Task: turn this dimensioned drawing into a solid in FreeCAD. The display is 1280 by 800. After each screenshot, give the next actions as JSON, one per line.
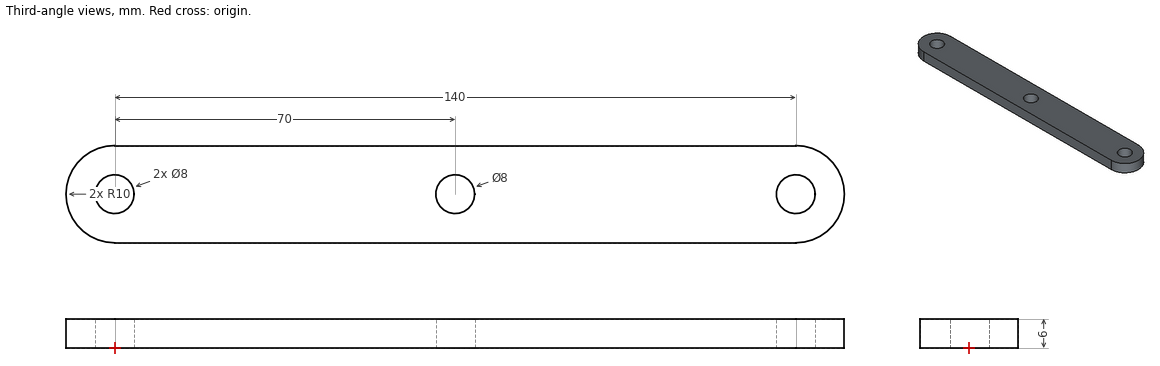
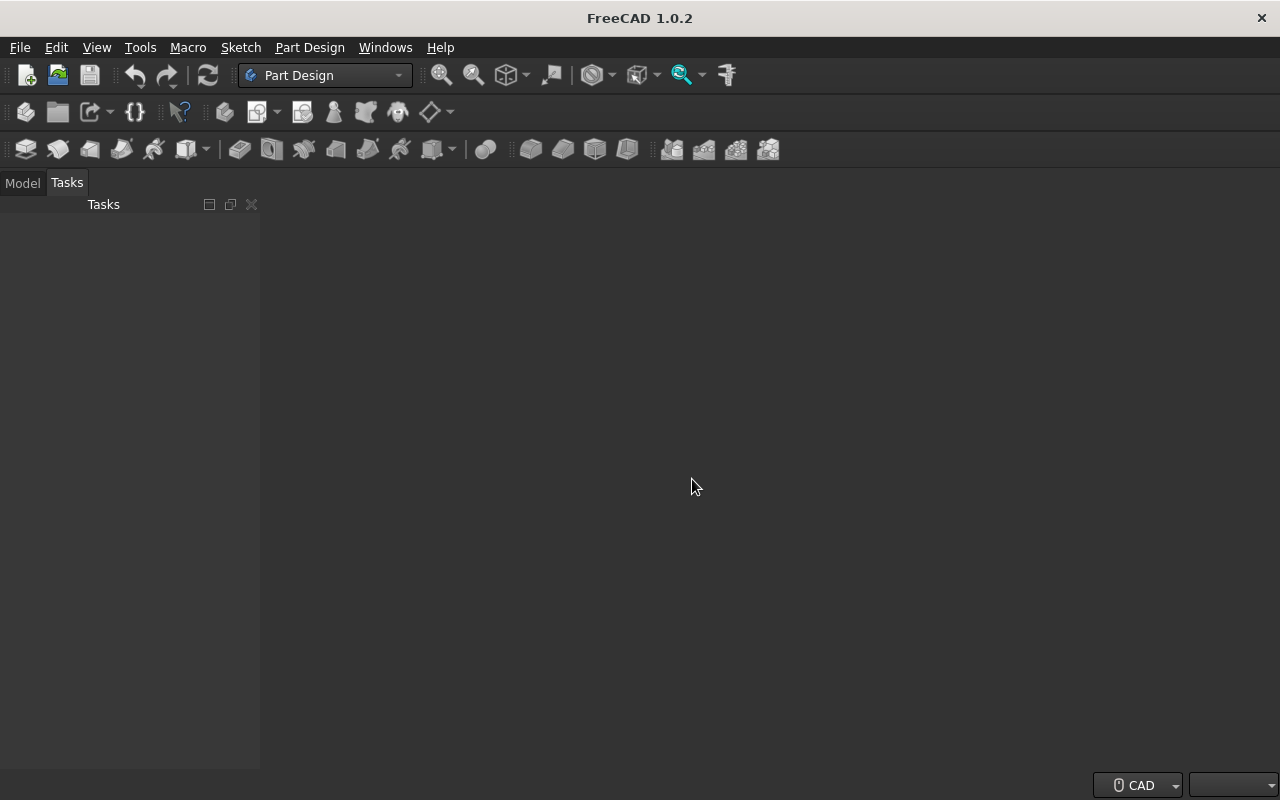
{"action": "left_click", "coordinate": [26, 76]}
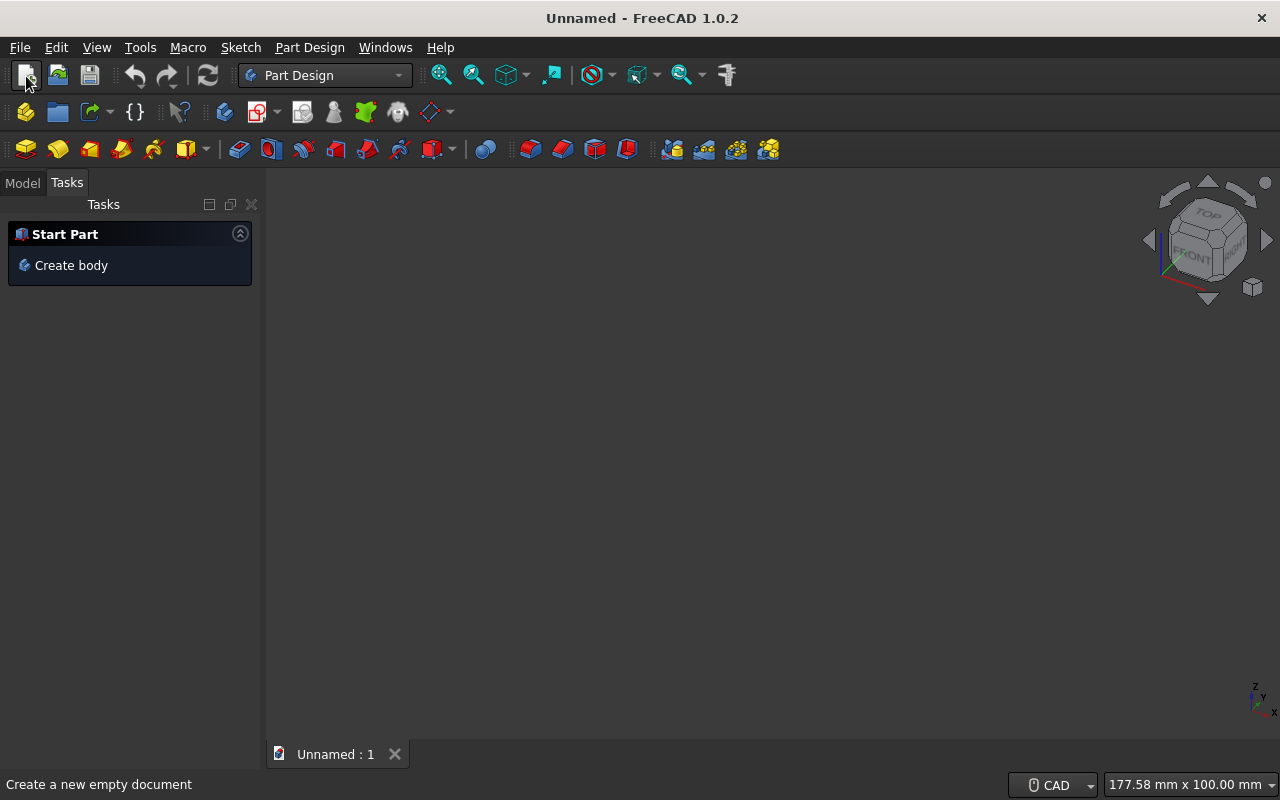
{"action": "left_click", "coordinate": [258, 112]}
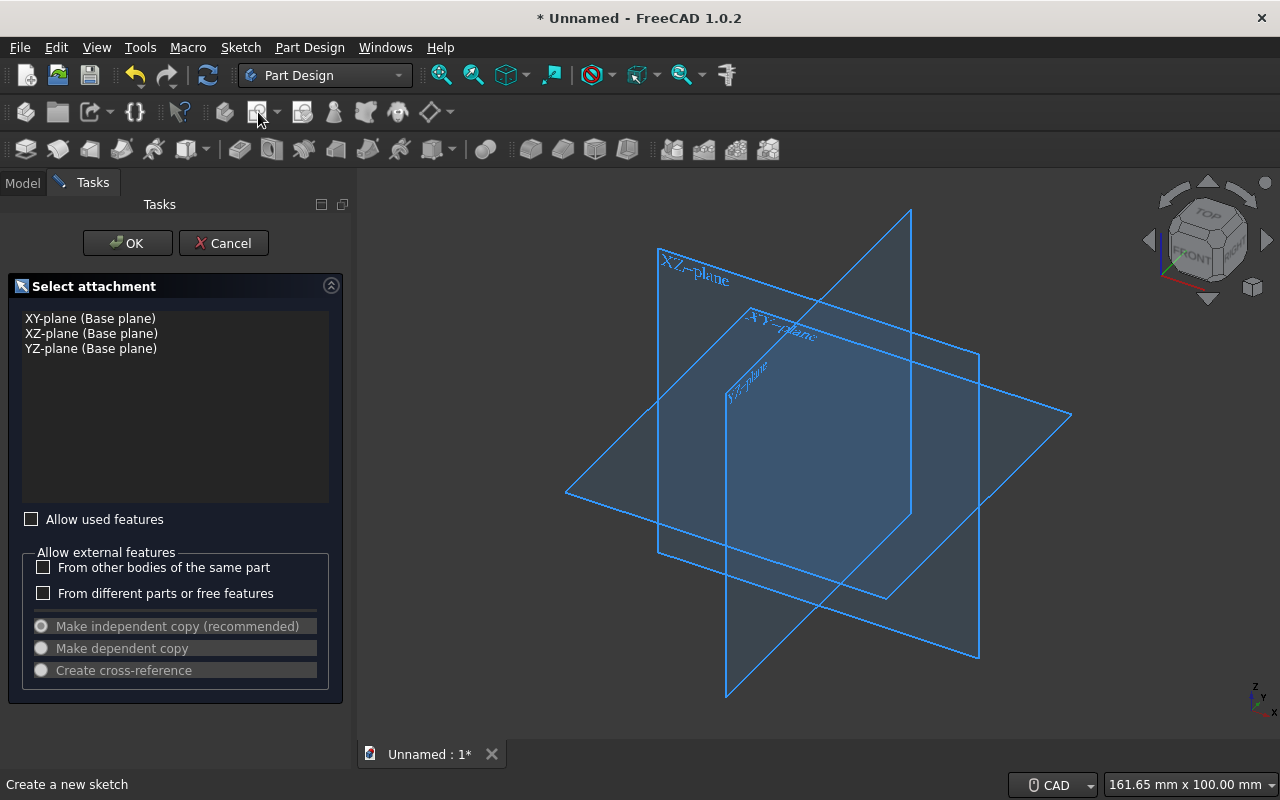
{"action": "left_click", "coordinate": [82, 318]}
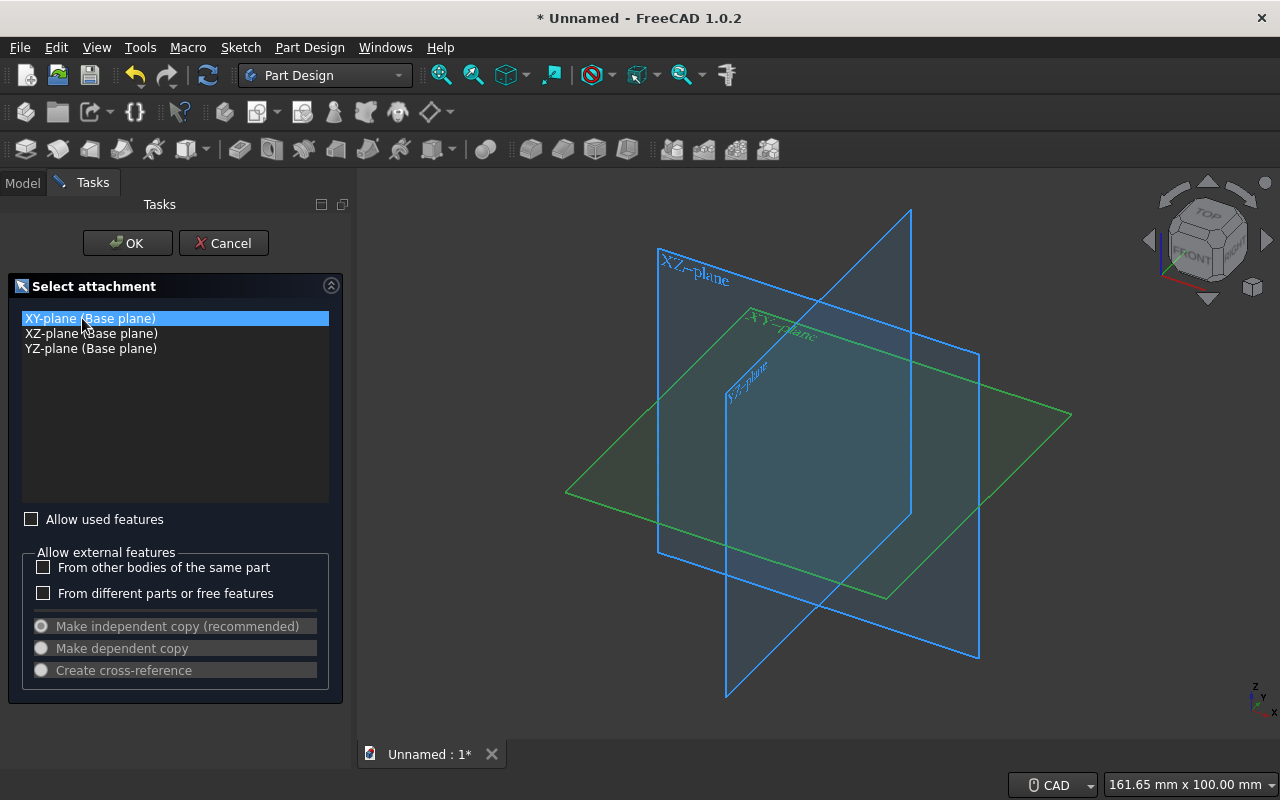
{"action": "left_click", "coordinate": [128, 243]}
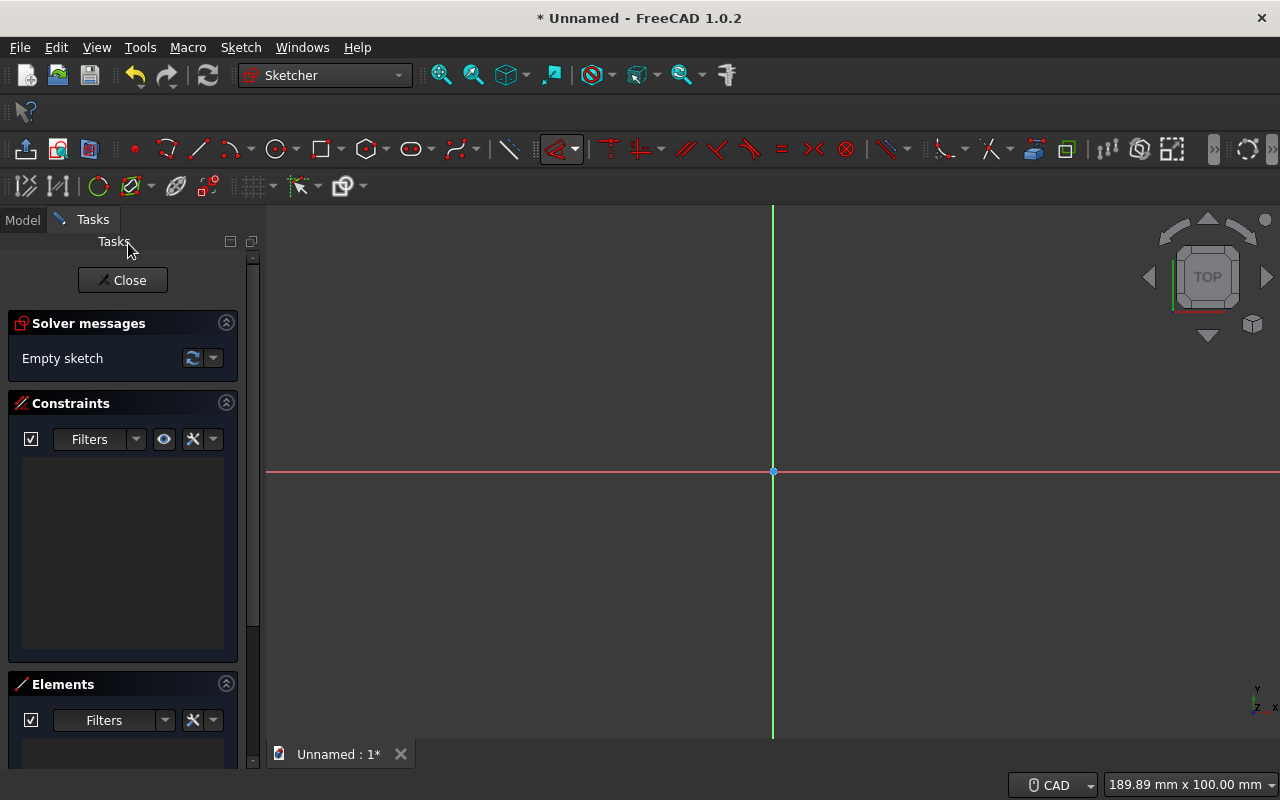
{"action": "scroll", "coordinate": [294, 472], "scroll_direction": "down", "scroll_amount": 3}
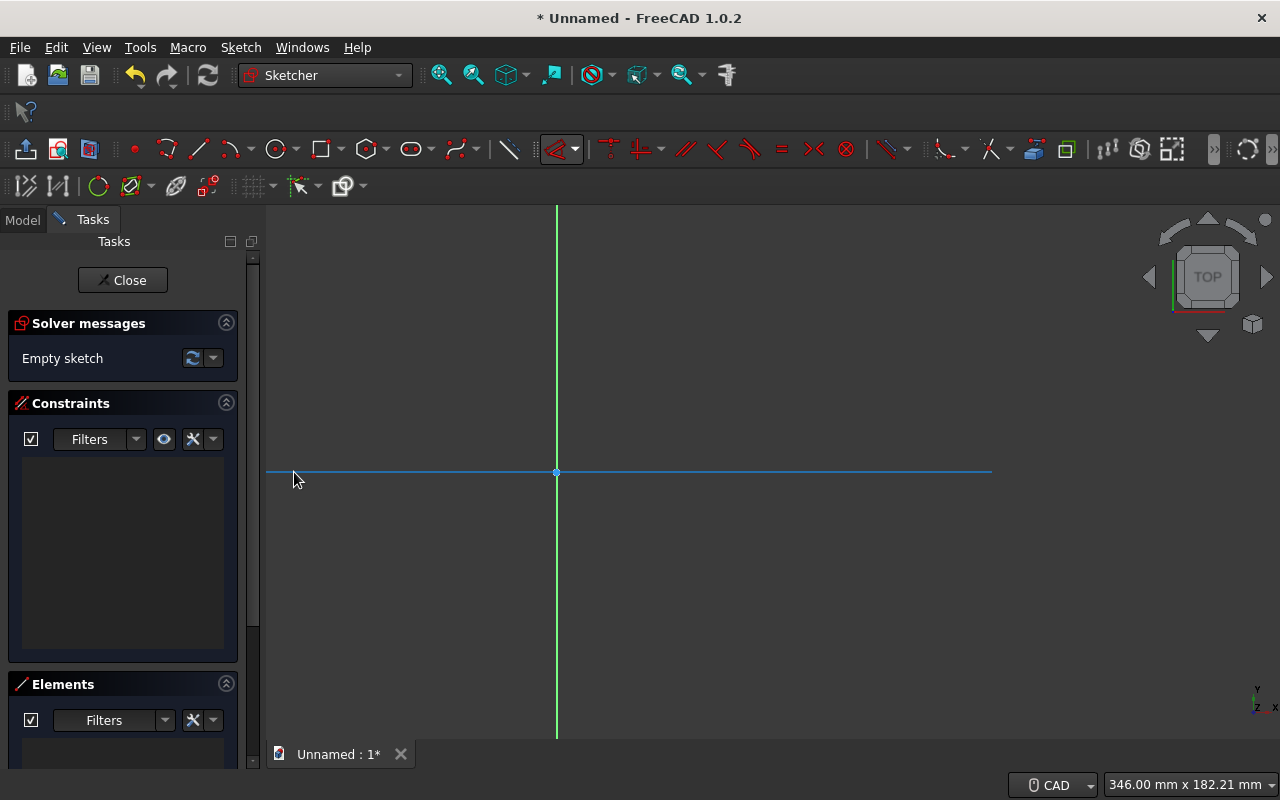
{"action": "key", "text": "g s"}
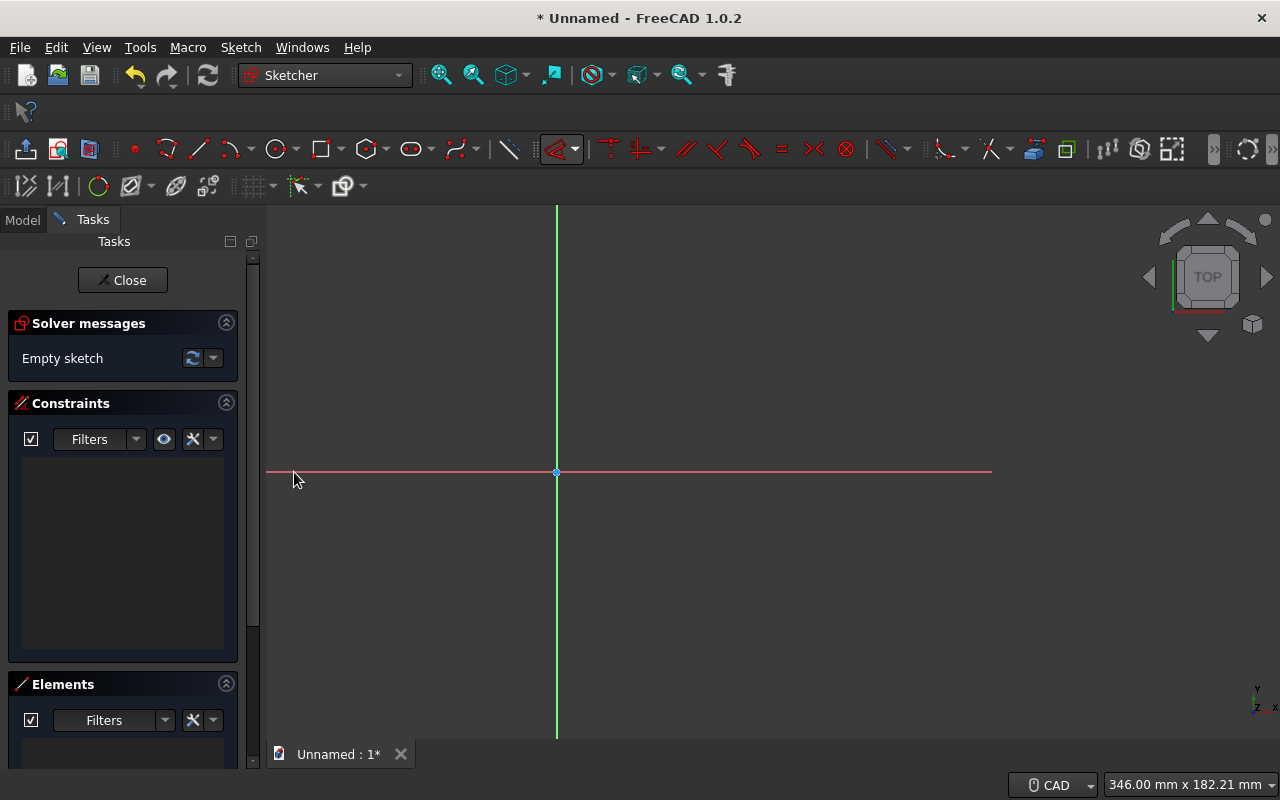
{"action": "left_click", "coordinate": [557, 472]}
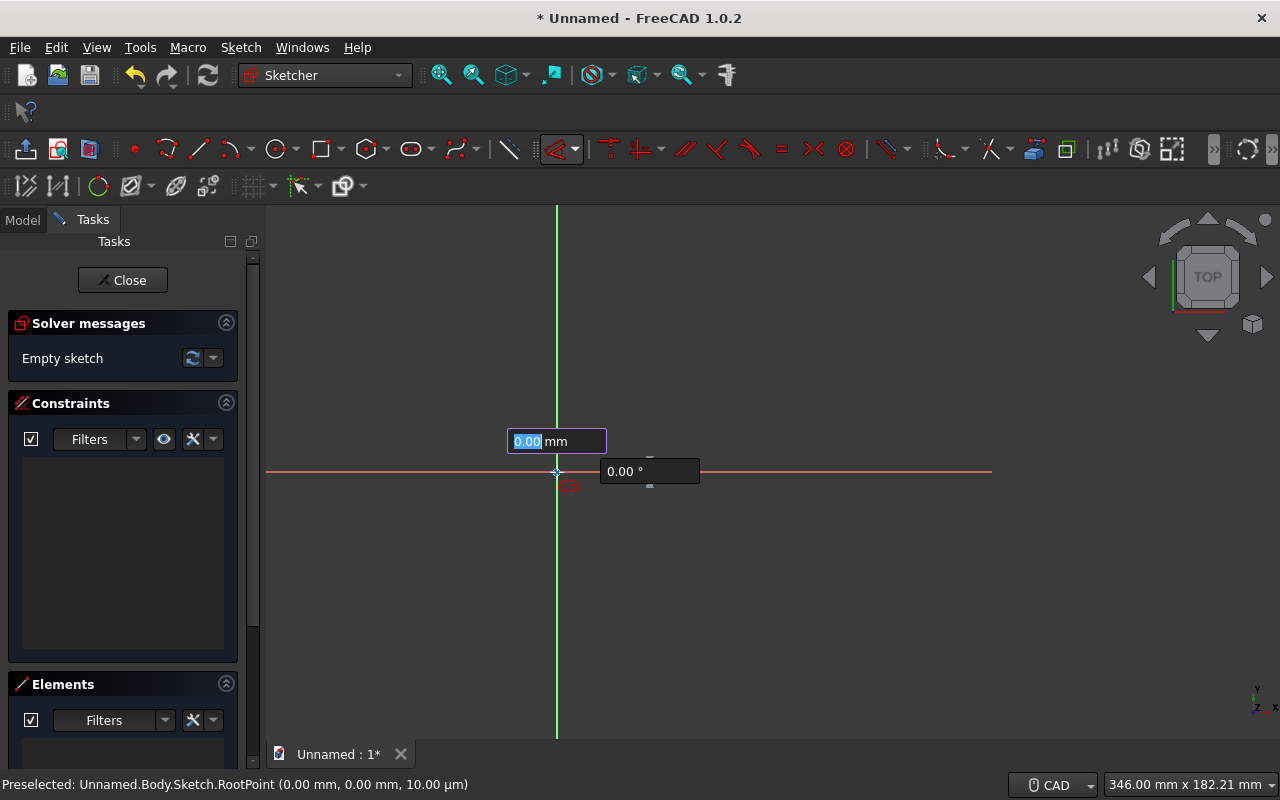
{"action": "left_click", "coordinate": [967, 463]}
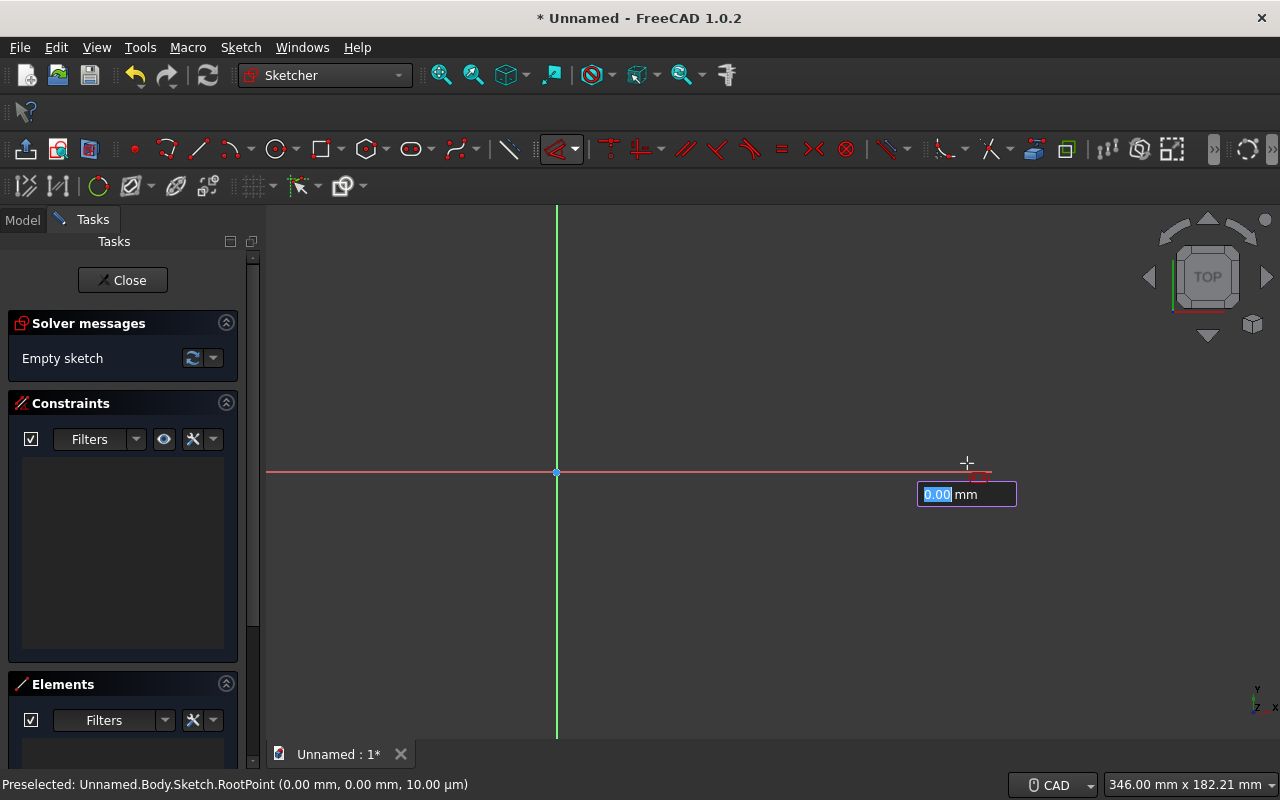
{"action": "left_click", "coordinate": [762, 443]}
{"action": "key", "text": "Escape"}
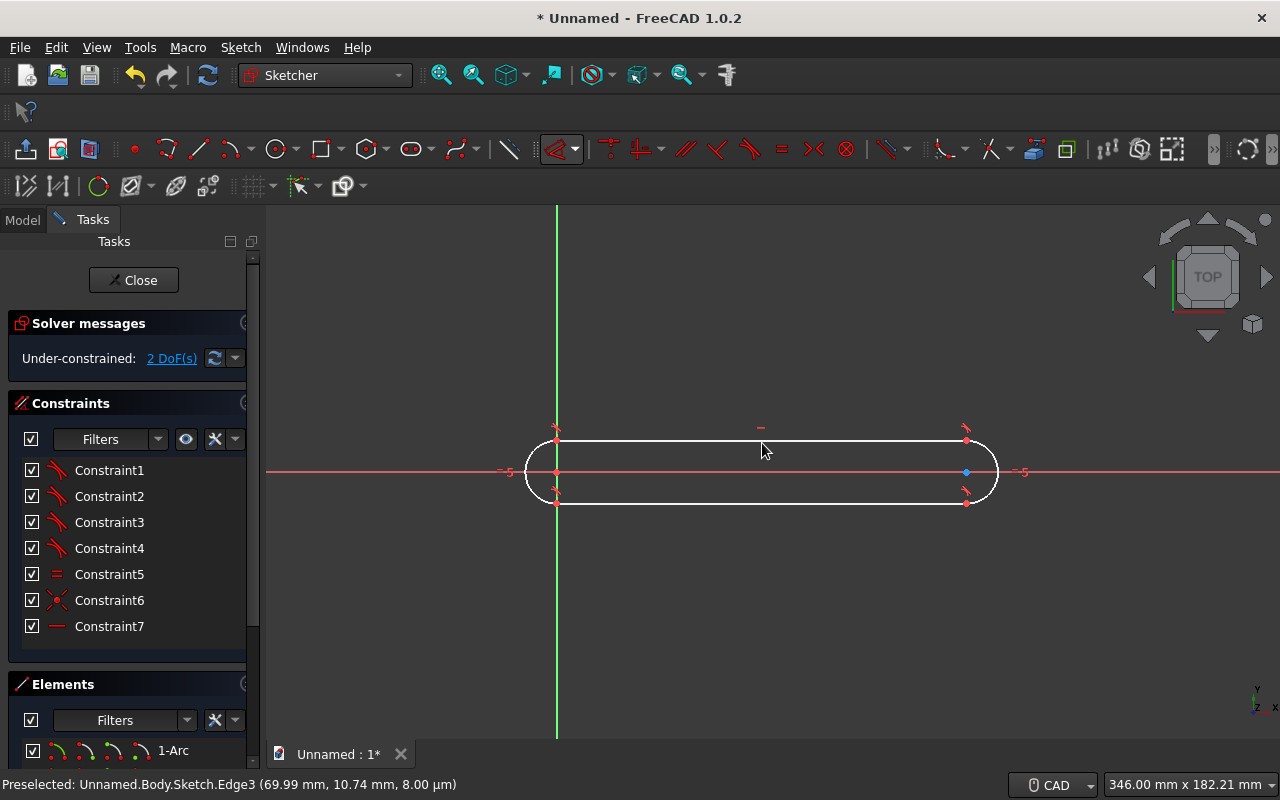
{"action": "scroll", "coordinate": [531, 454], "scroll_direction": "up", "scroll_amount": 2}